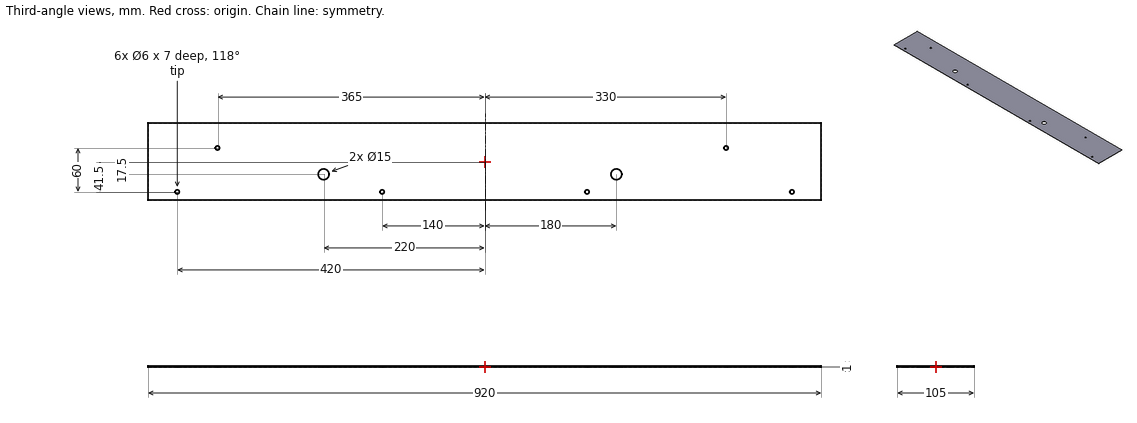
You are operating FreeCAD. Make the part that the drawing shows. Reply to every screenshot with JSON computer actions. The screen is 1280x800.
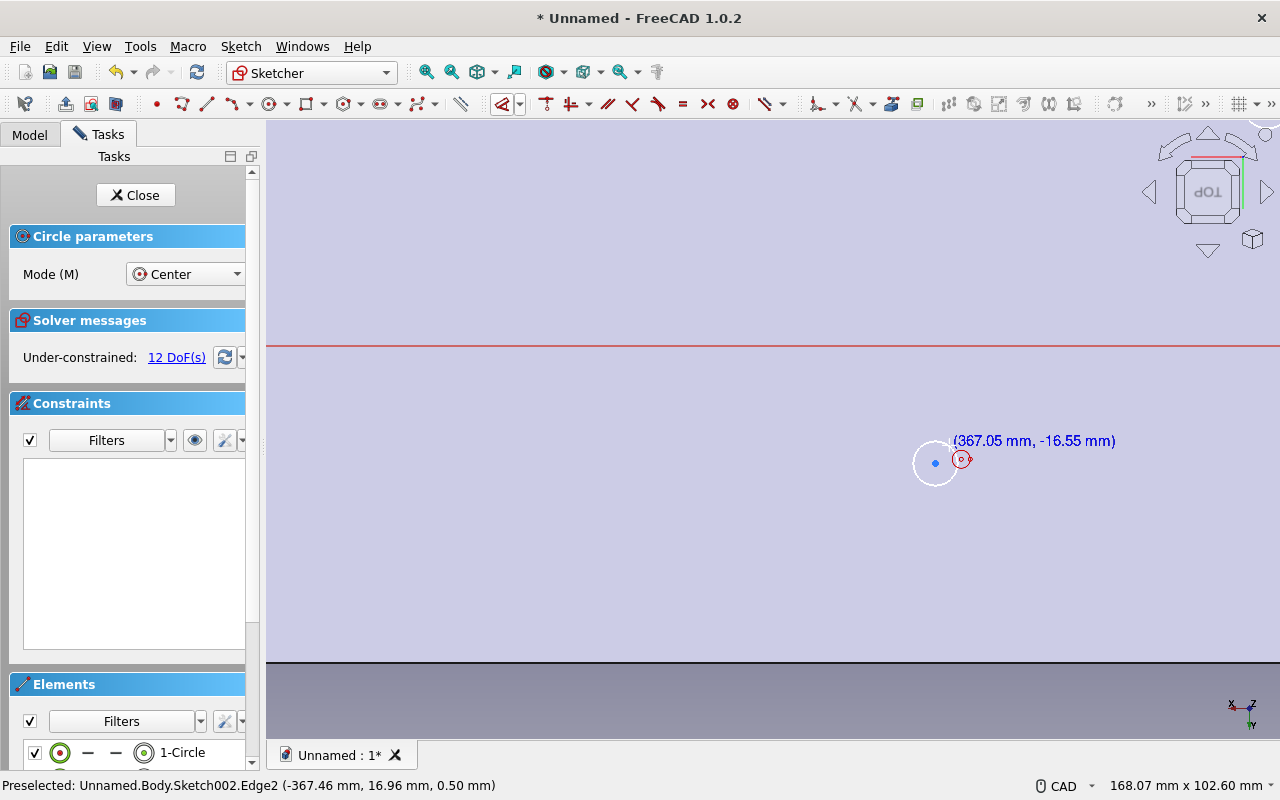
{"action": "scroll", "coordinate": [950, 449], "scroll_direction": "down", "scroll_amount": 11}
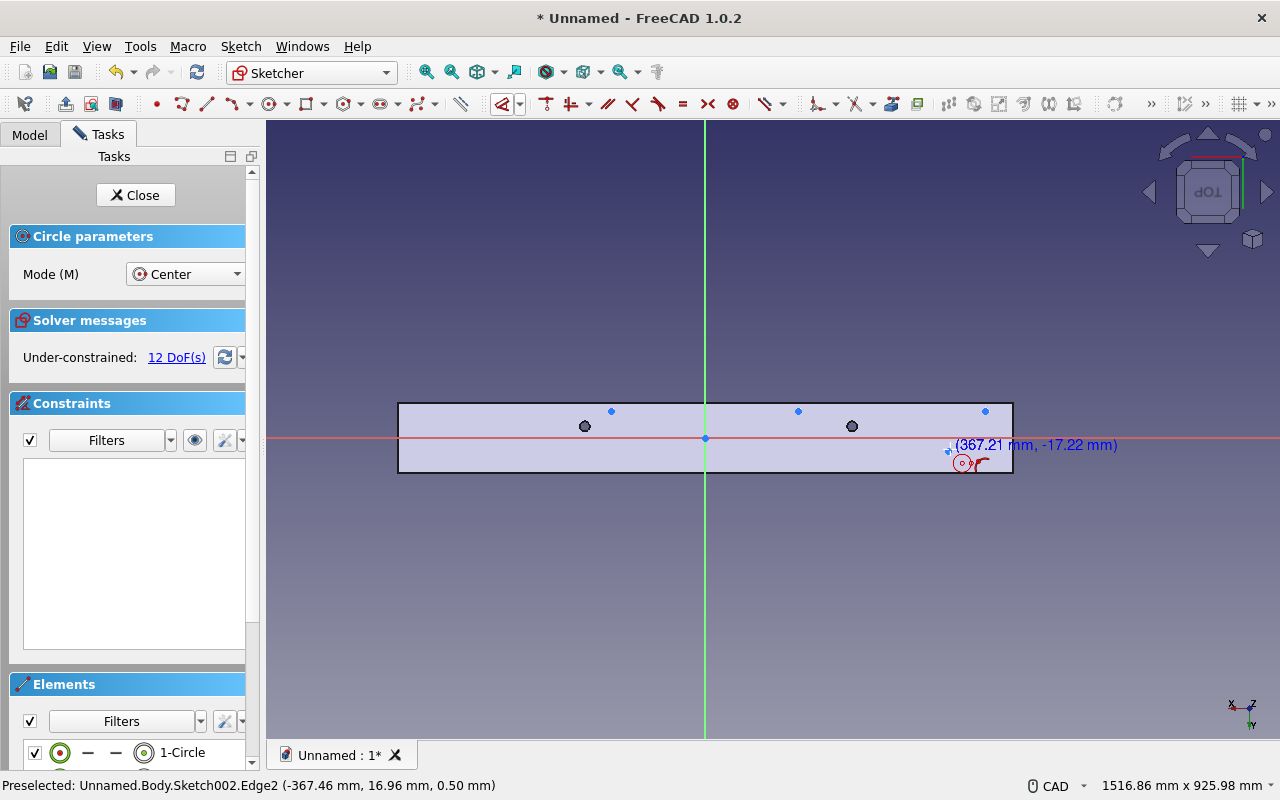
{"action": "scroll", "coordinate": [485, 450], "scroll_direction": "up", "scroll_amount": 13}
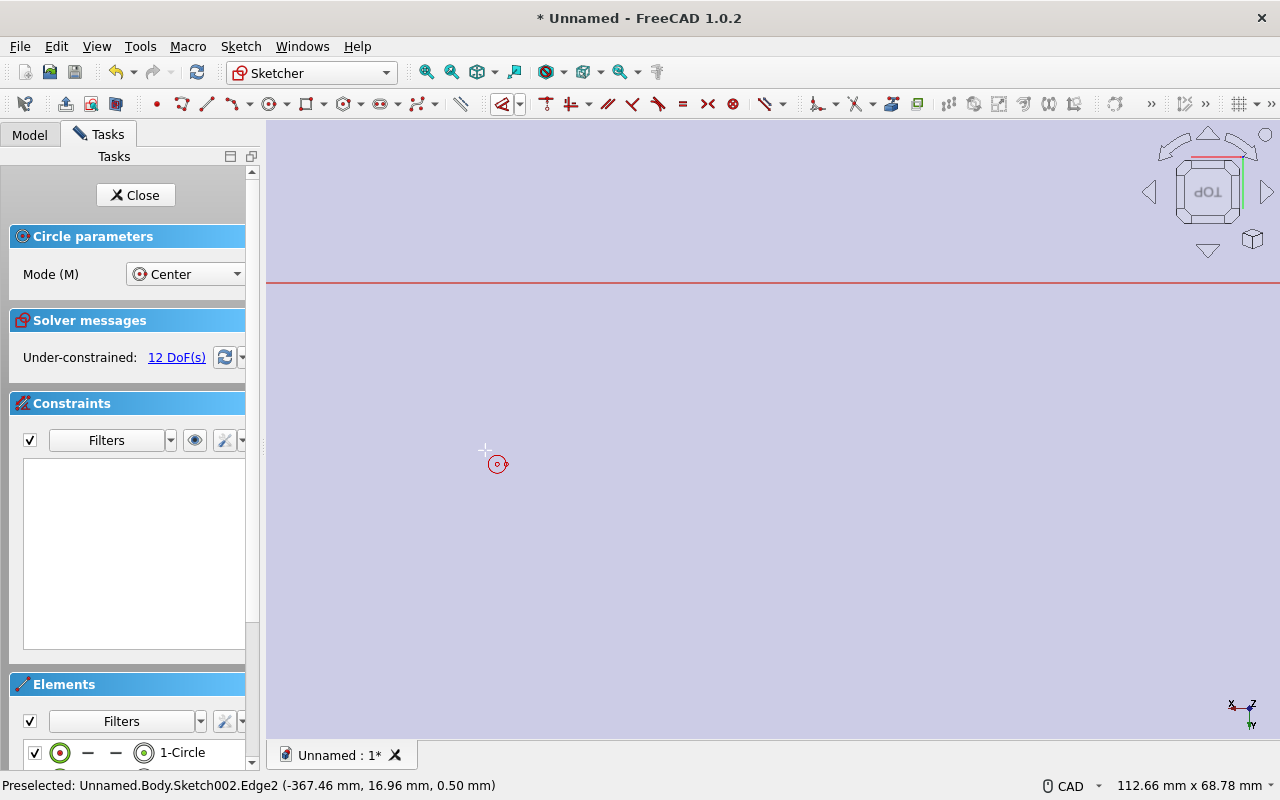
{"action": "scroll", "coordinate": [485, 450], "scroll_direction": "down", "scroll_amount": 13}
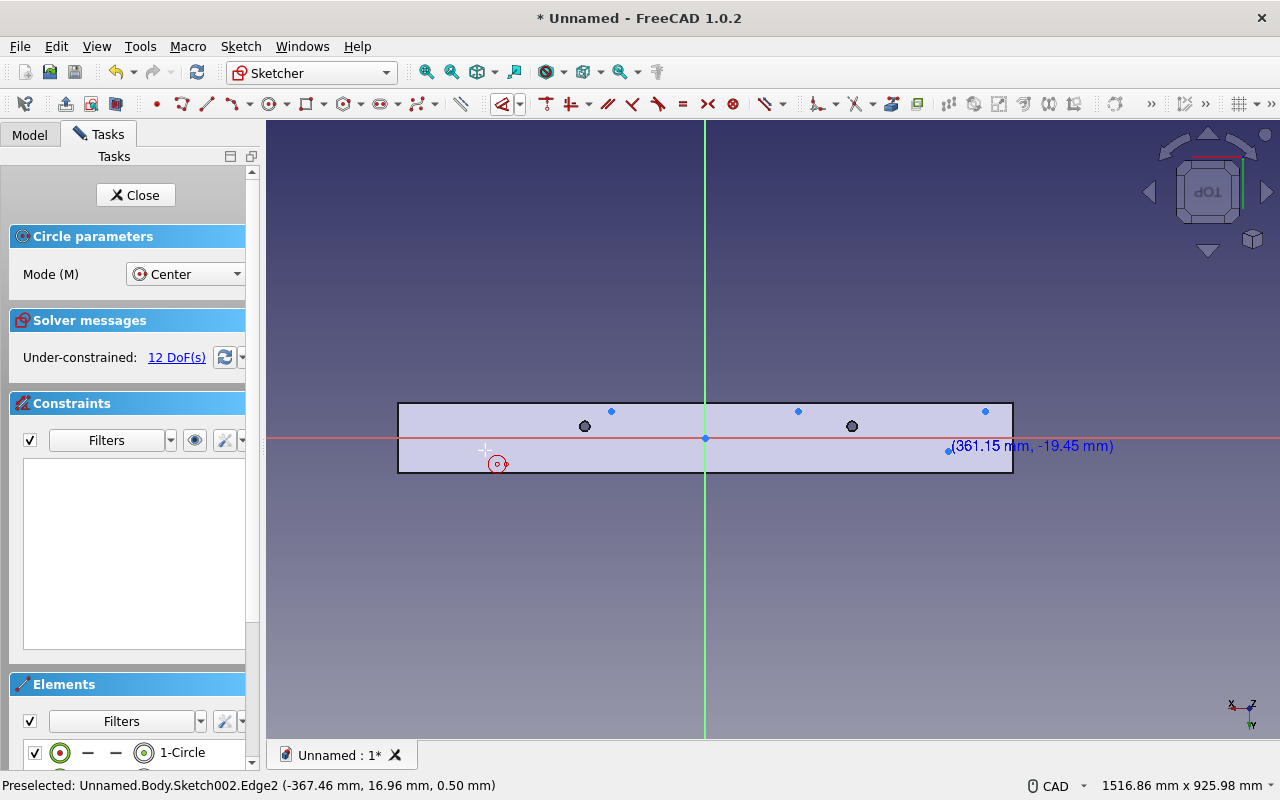
{"action": "scroll", "coordinate": [485, 450], "scroll_direction": "up", "scroll_amount": 2}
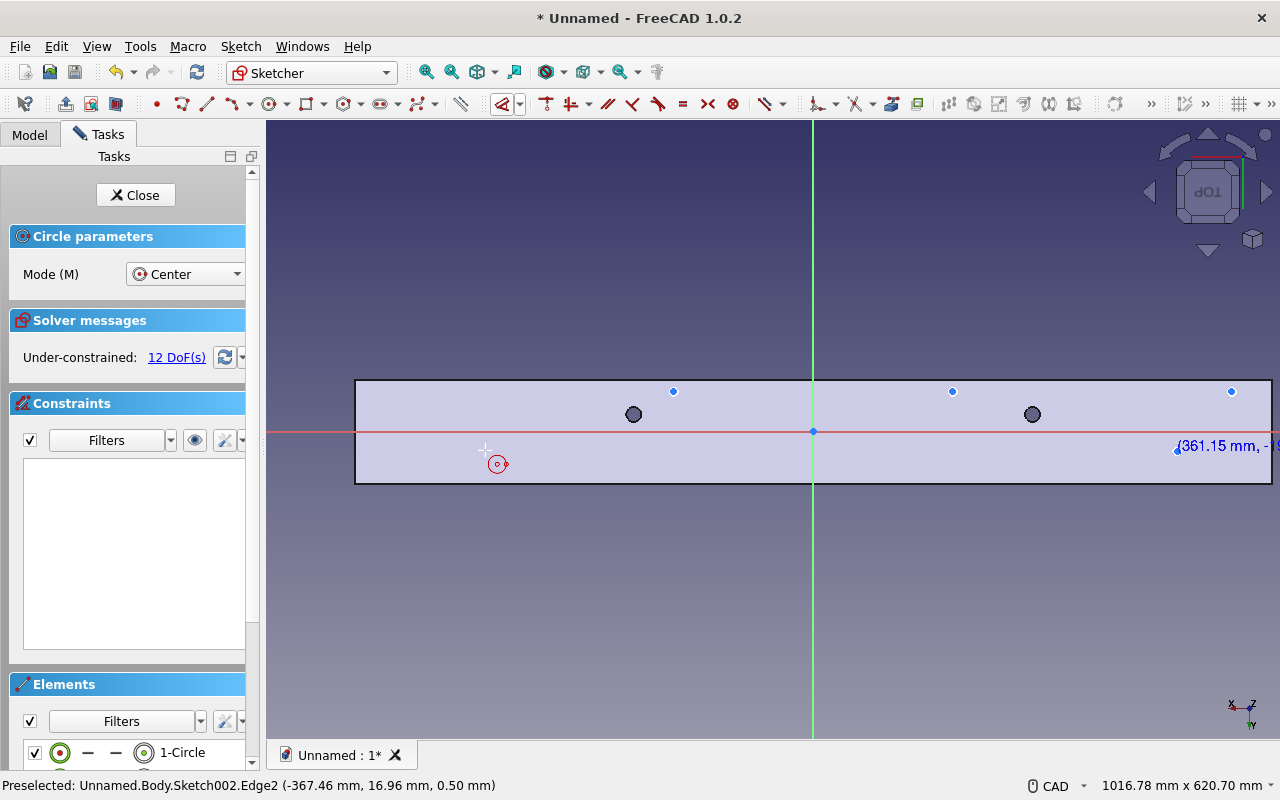
{"action": "left_click", "coordinate": [484, 450]}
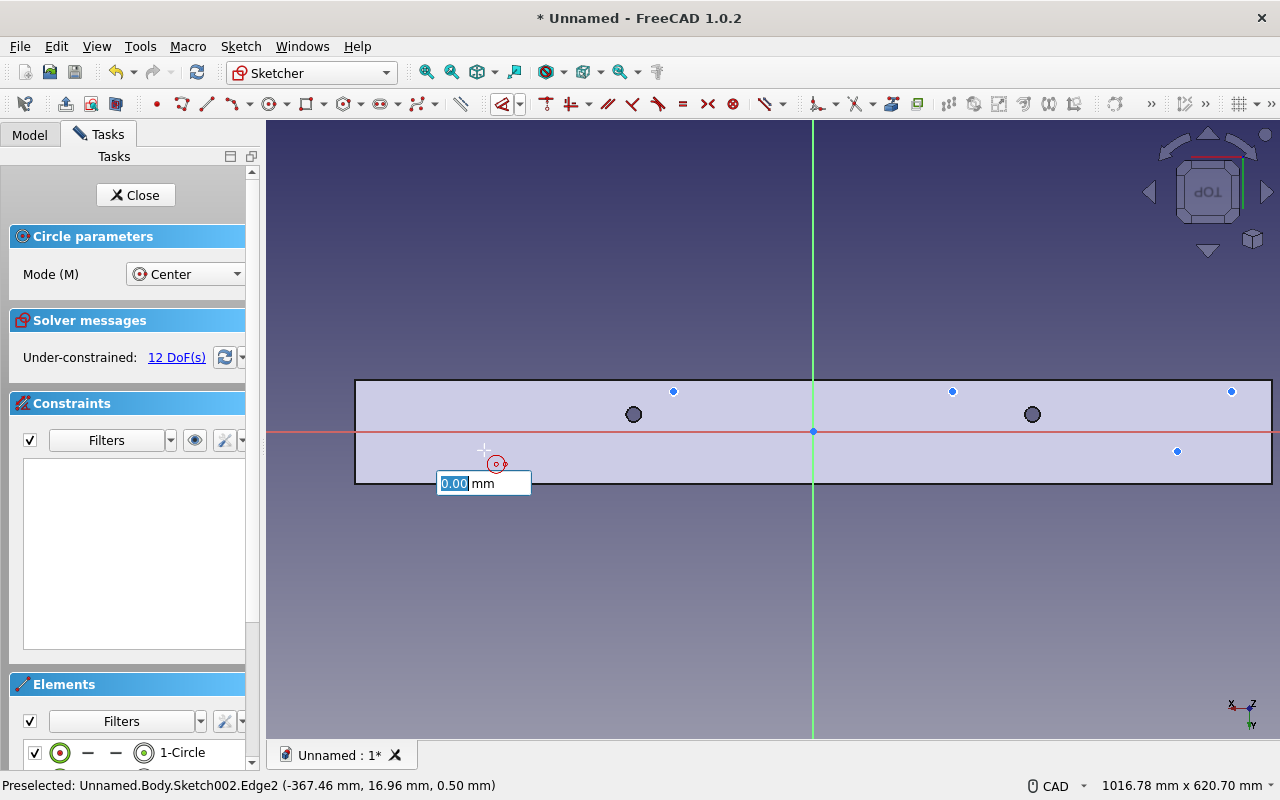
{"action": "scroll", "coordinate": [486, 448], "scroll_direction": "up", "scroll_amount": 9}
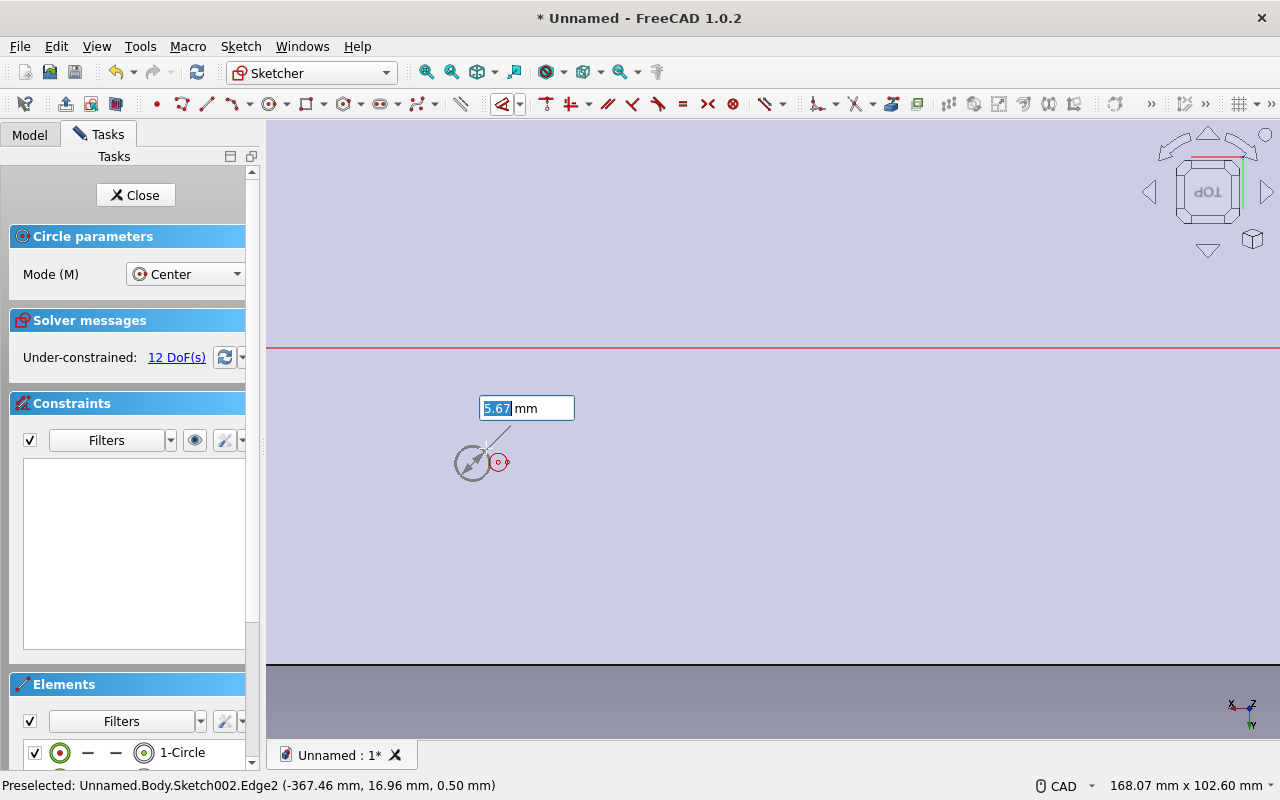
{"action": "left_click", "coordinate": [487, 447]}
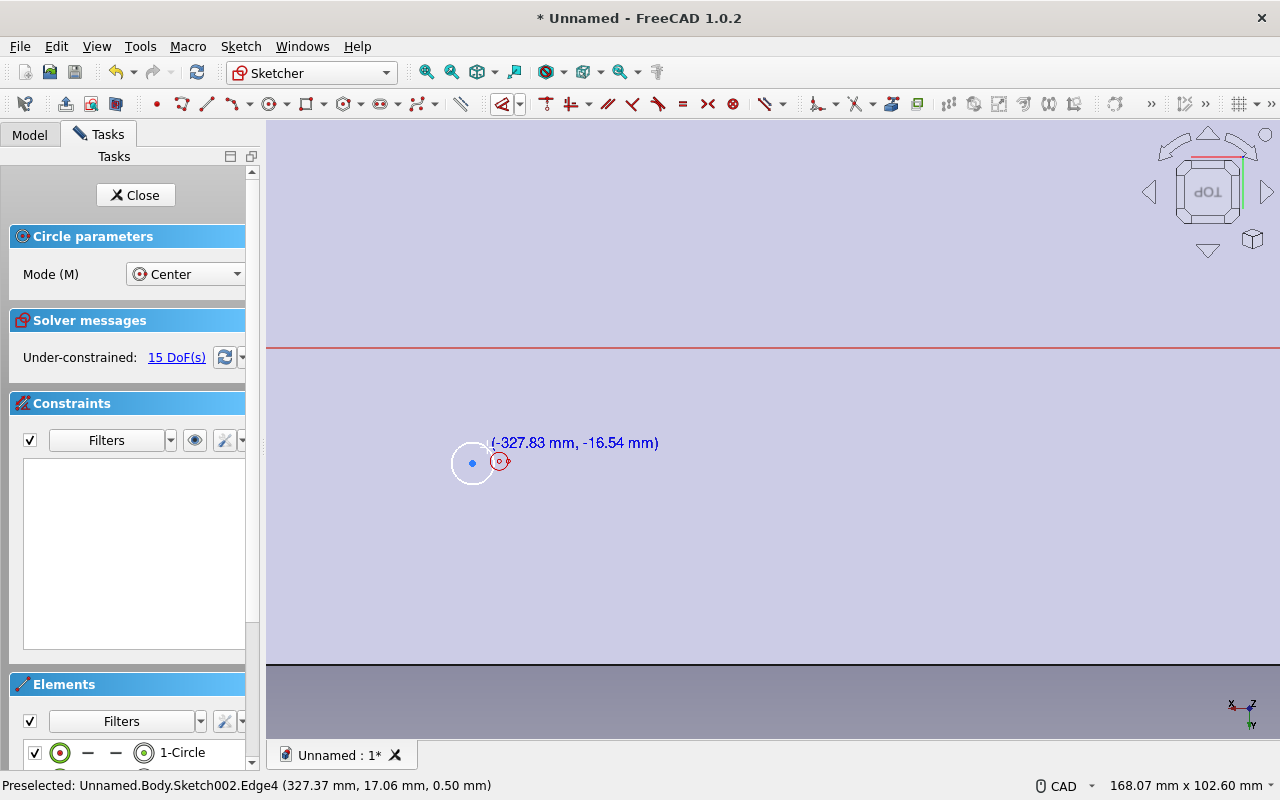
{"action": "scroll", "coordinate": [485, 448], "scroll_direction": "down", "scroll_amount": 11}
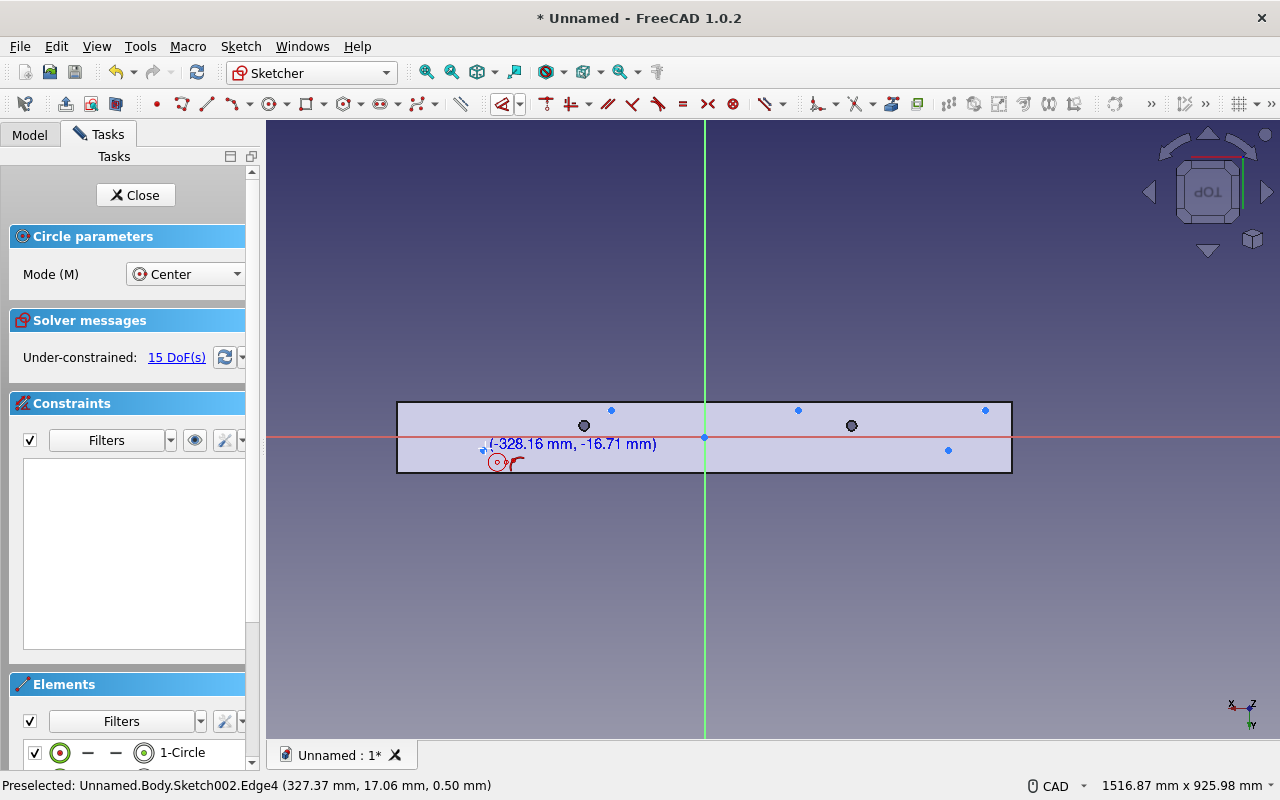
{"action": "scroll", "coordinate": [424, 410], "scroll_direction": "up", "scroll_amount": 13}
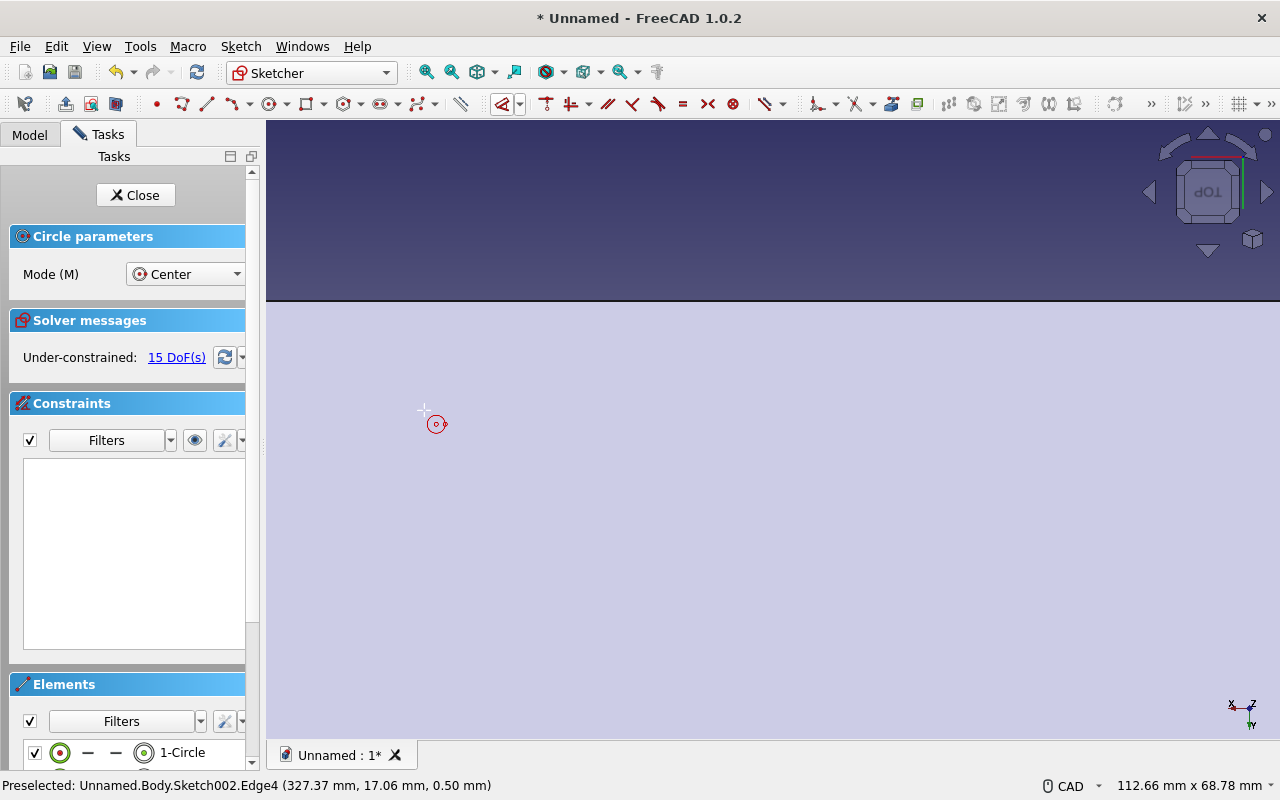
{"action": "scroll", "coordinate": [424, 410], "scroll_direction": "down", "scroll_amount": 13}